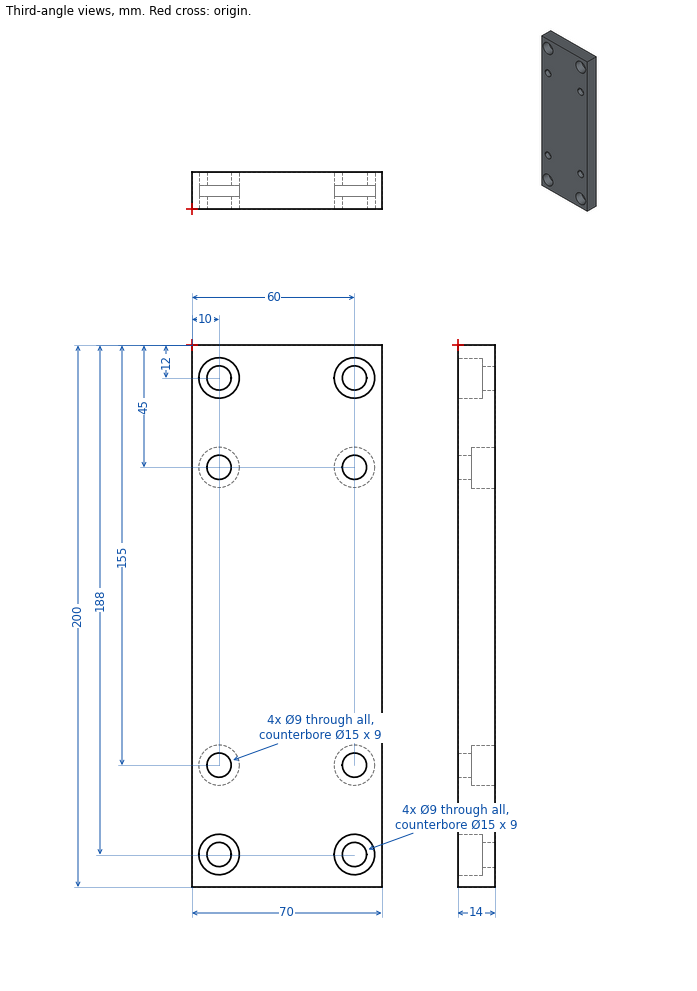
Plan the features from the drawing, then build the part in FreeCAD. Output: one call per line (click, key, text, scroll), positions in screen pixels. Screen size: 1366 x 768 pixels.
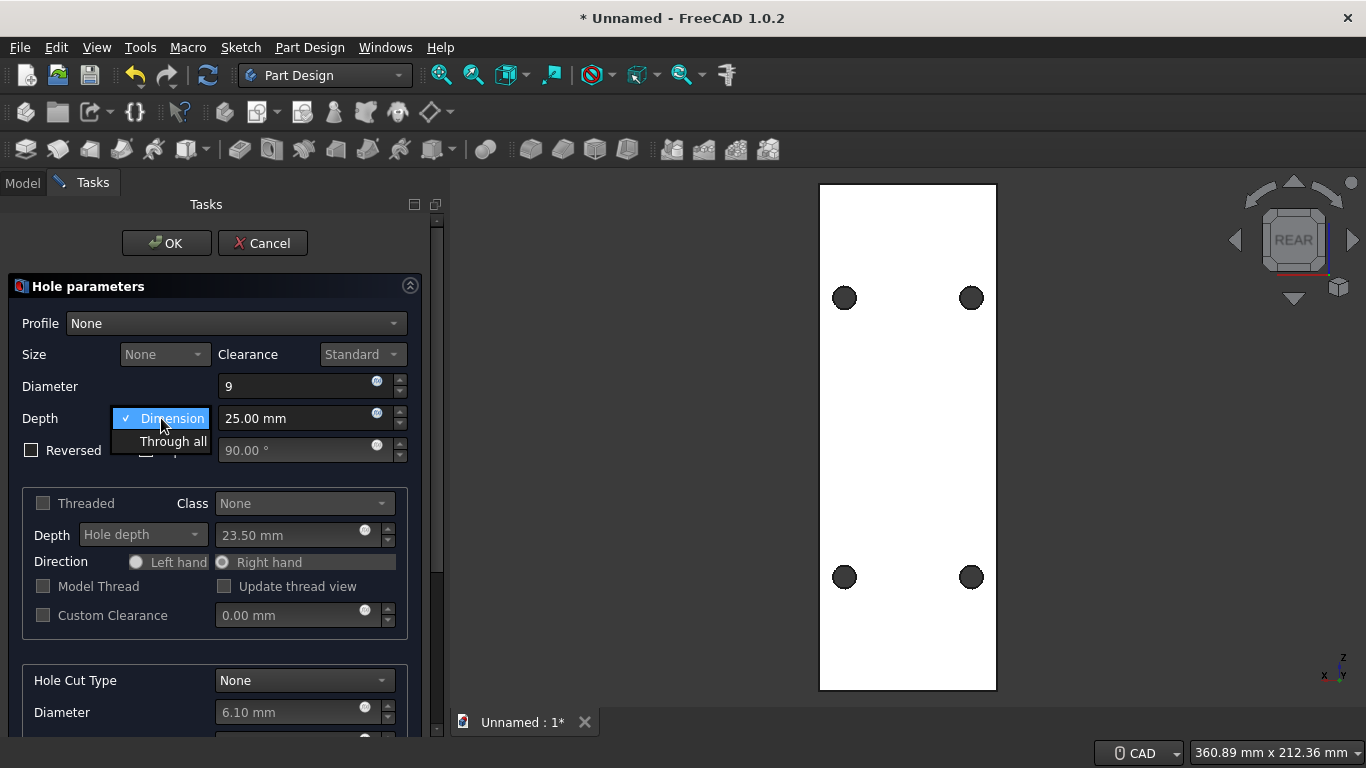
click(160, 442)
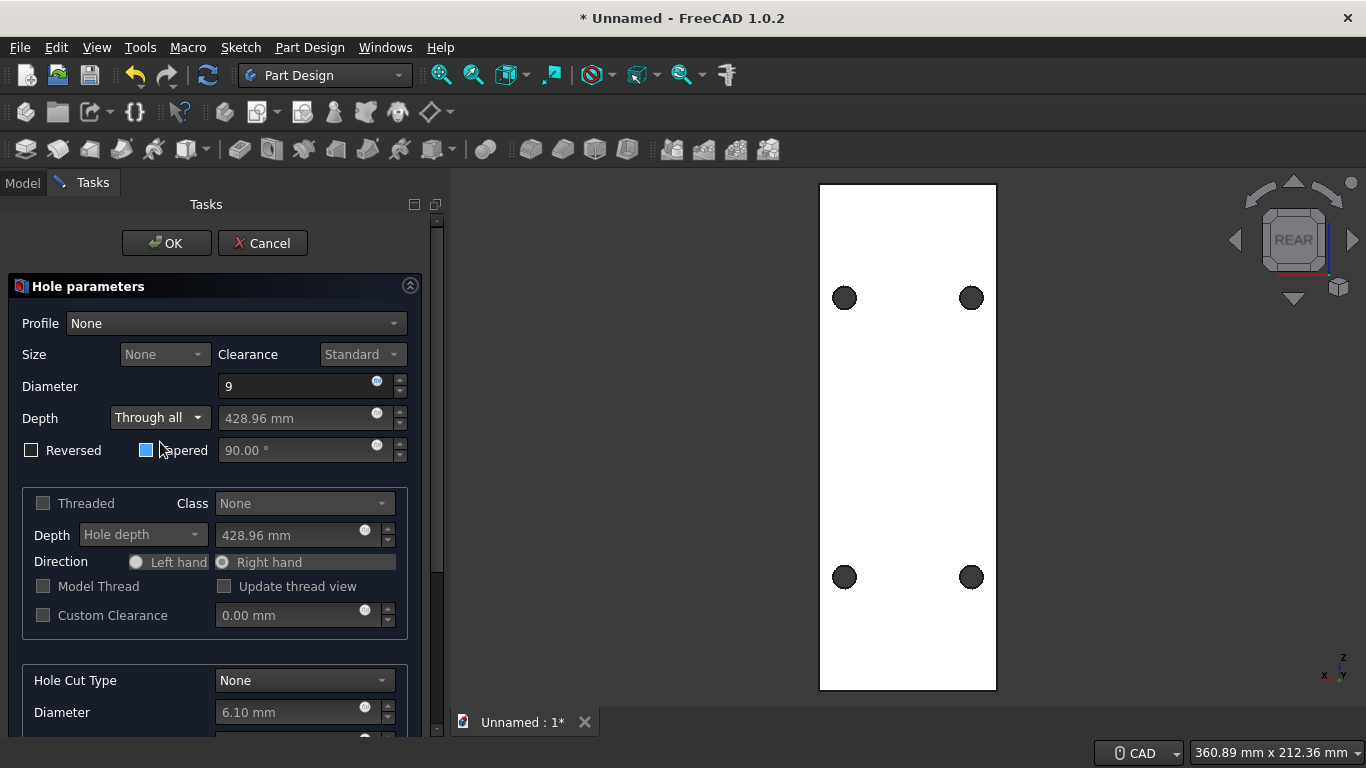
click(306, 680)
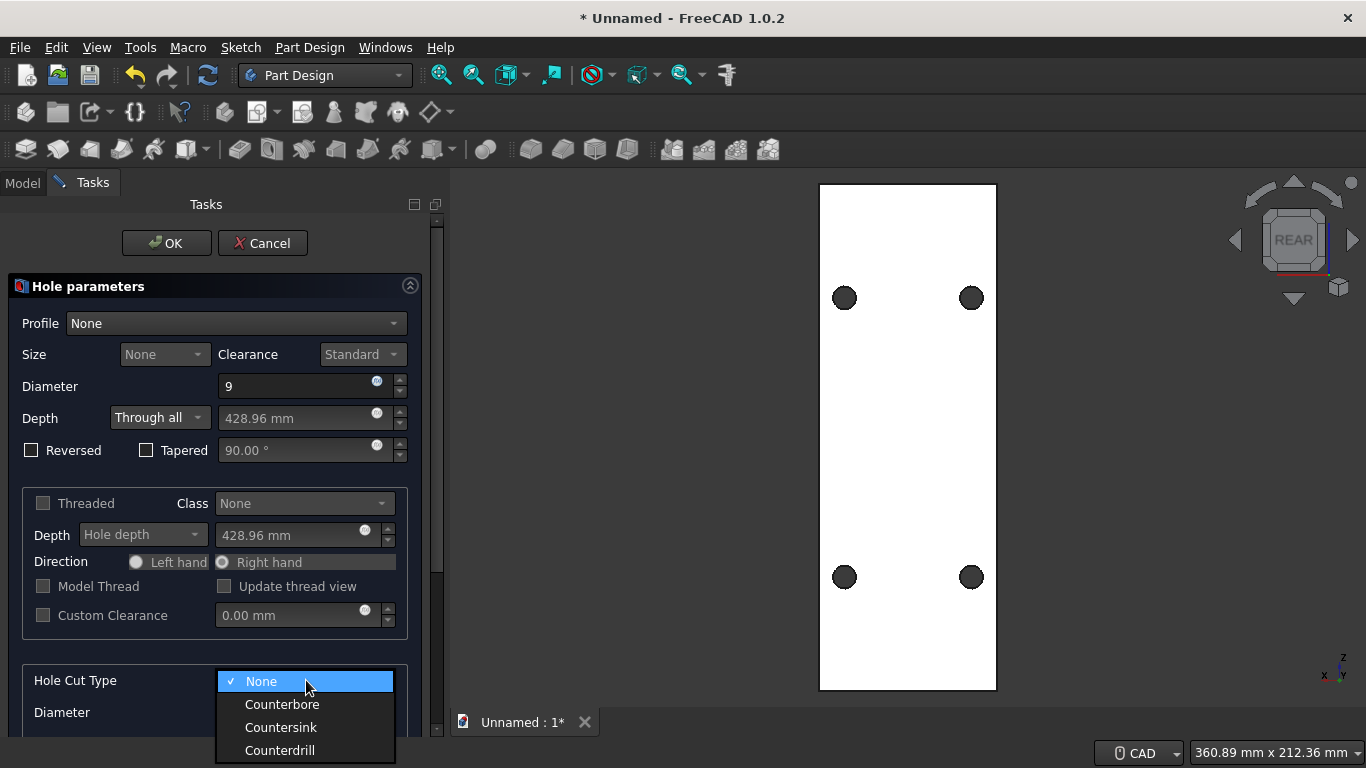
click(304, 704)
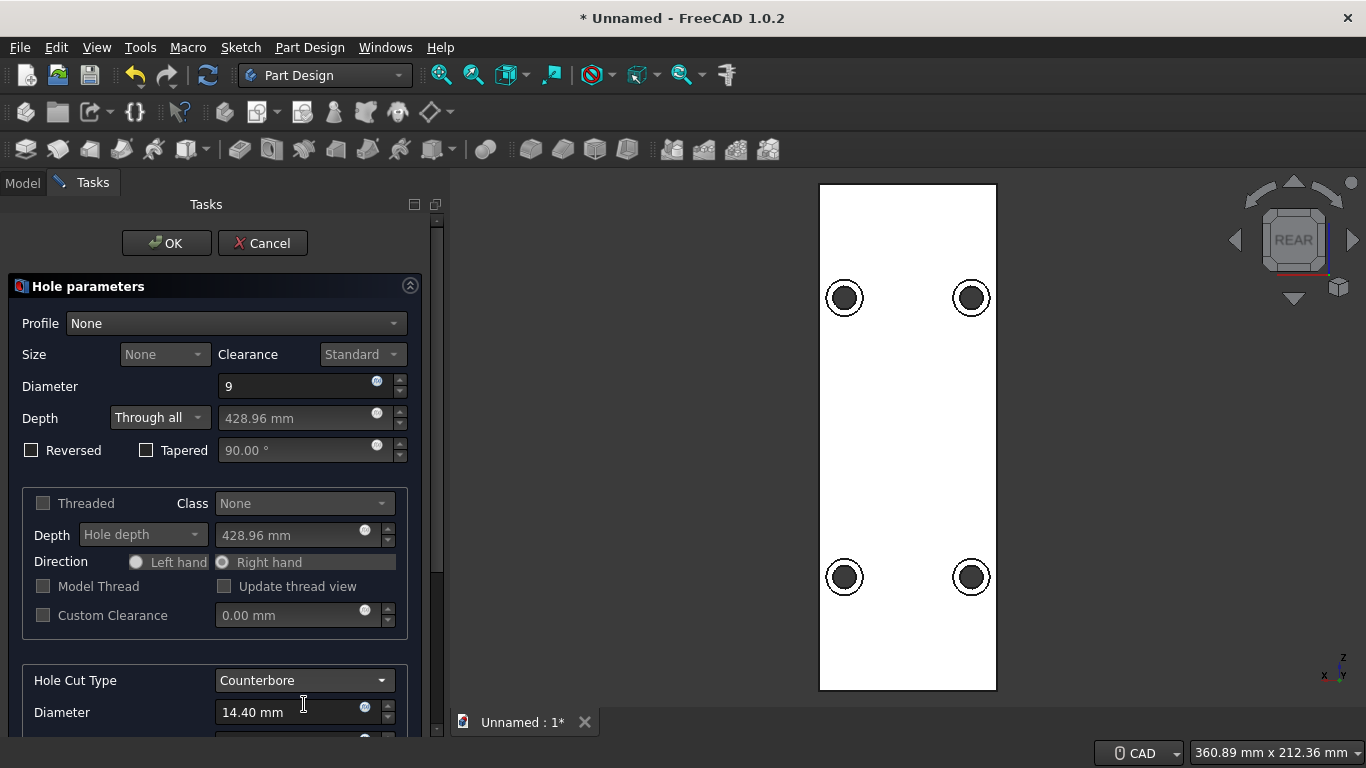
triple_click(298, 712)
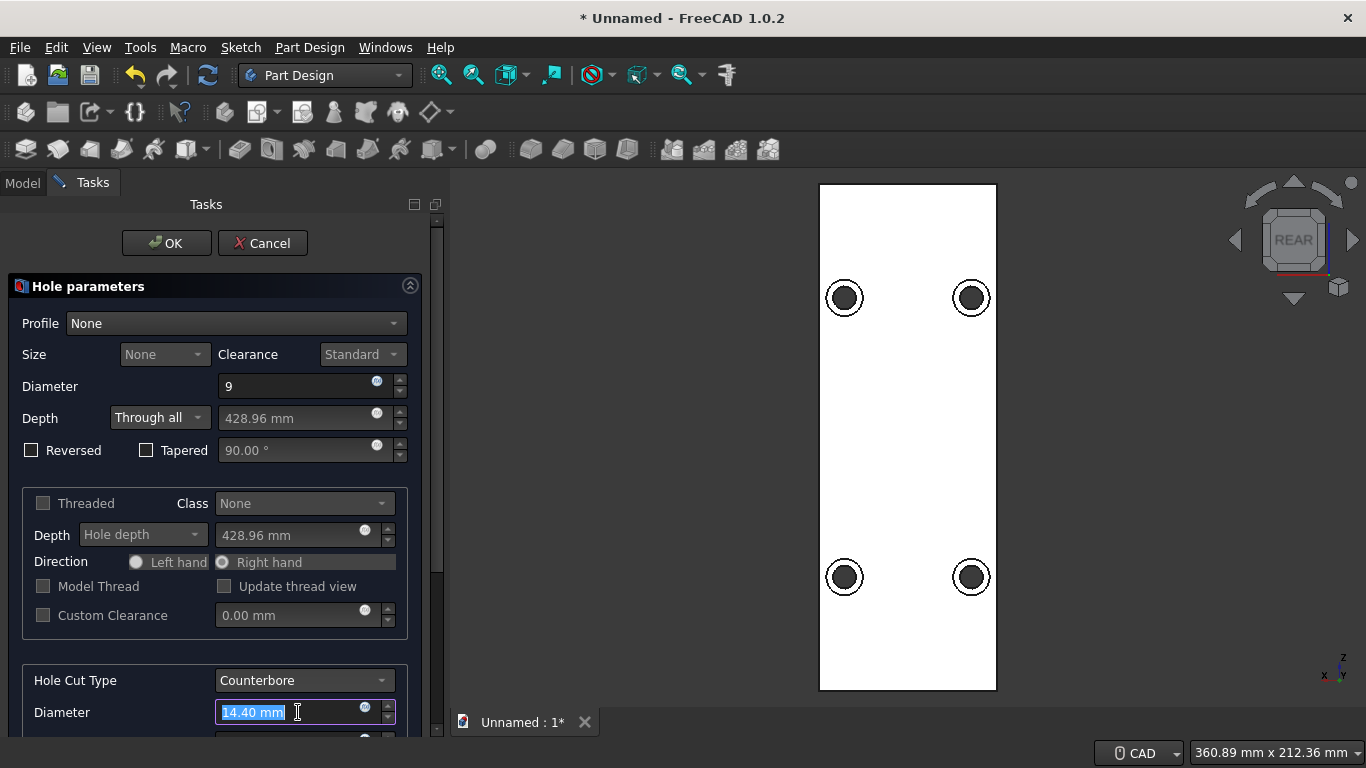
text(15)
key(Tab)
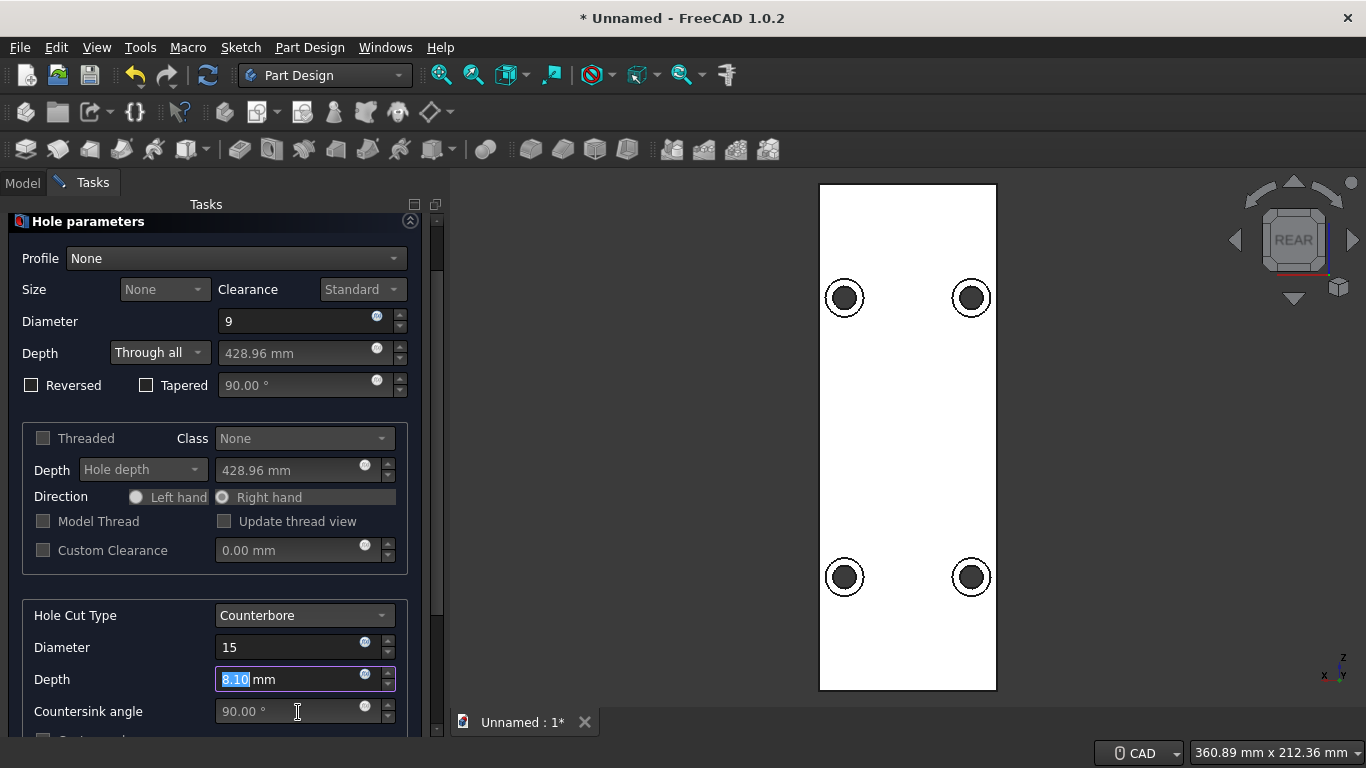
text(9)
key(Tab)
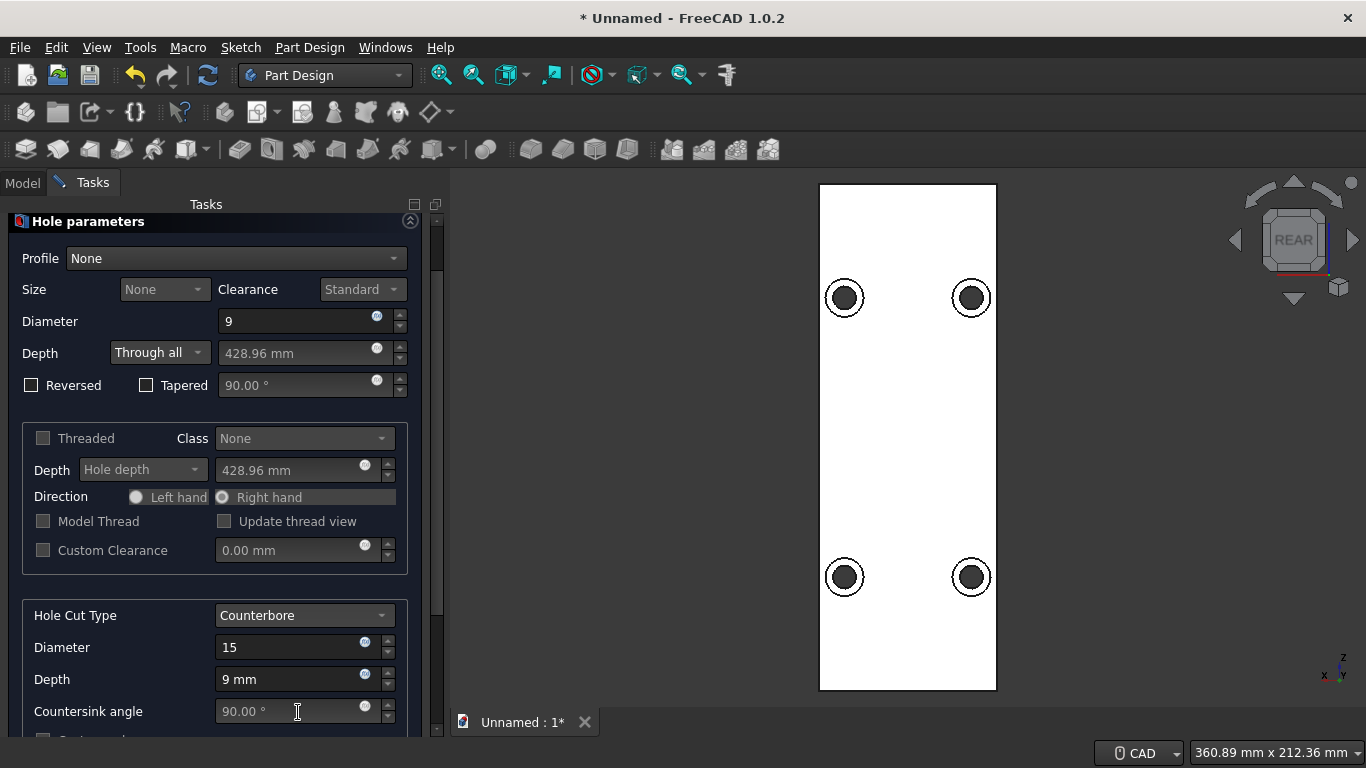
scroll(437, 475, up, 2)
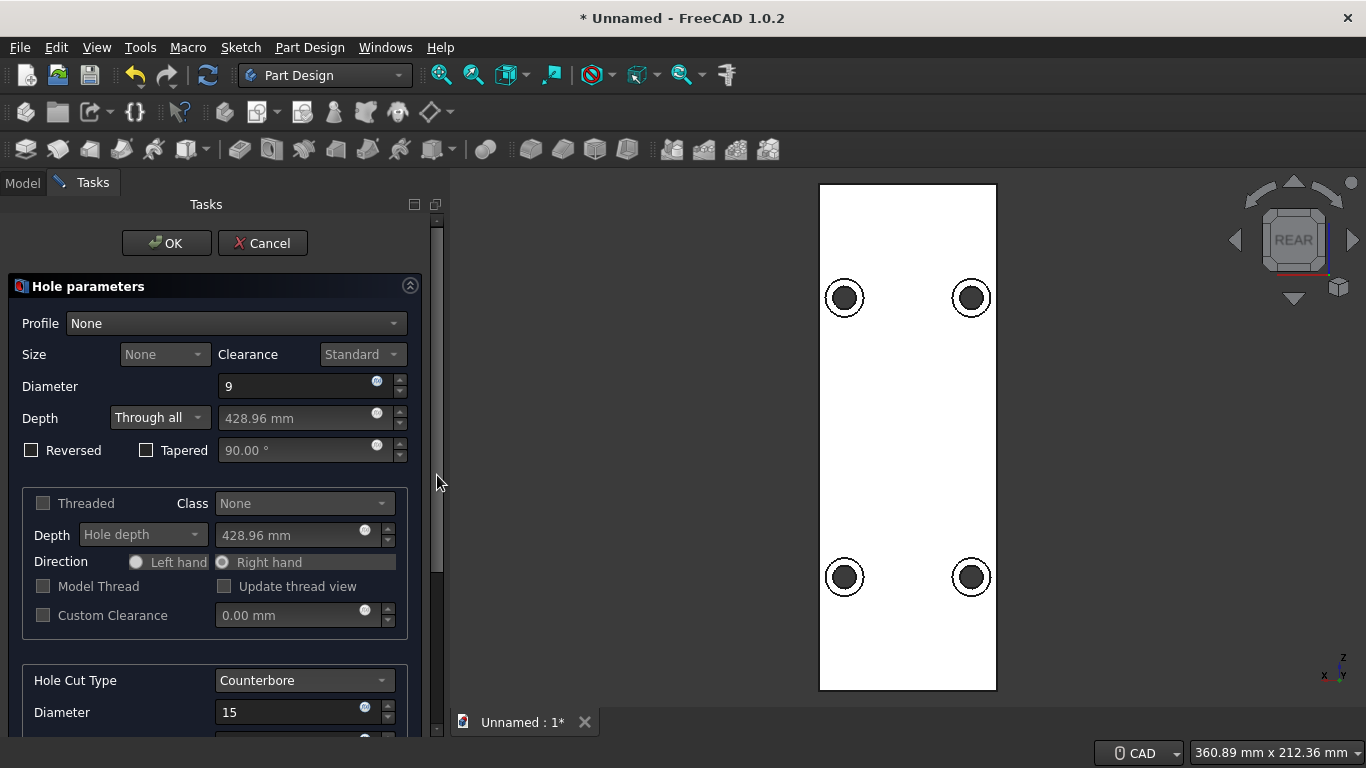
click(167, 243)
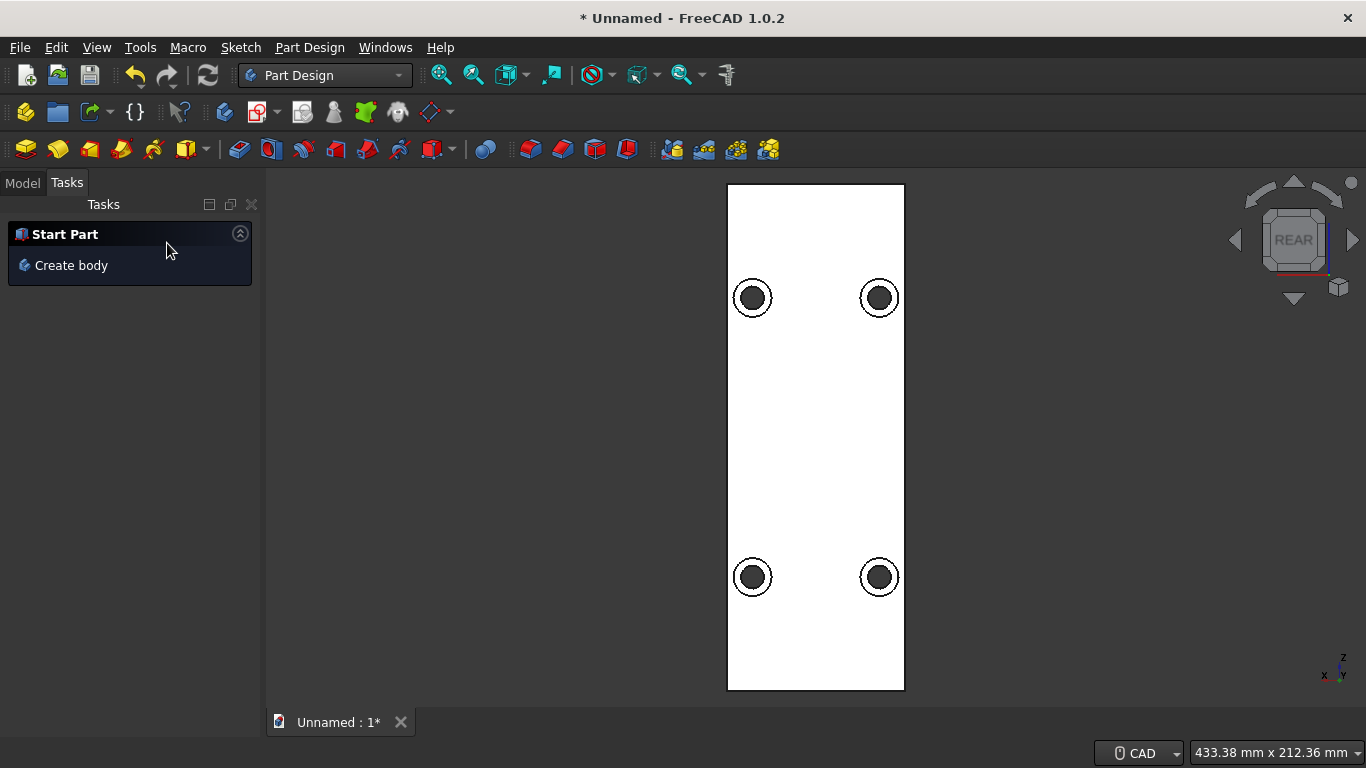
key(0)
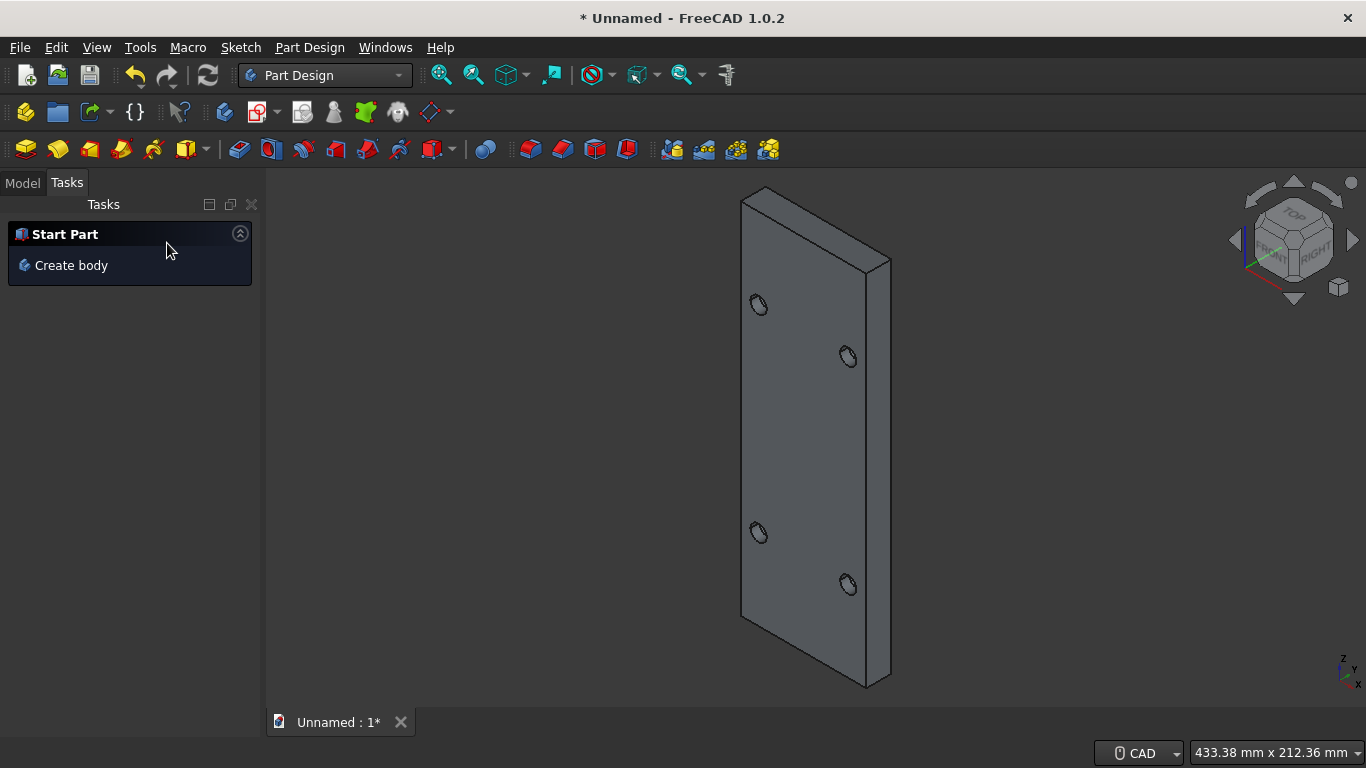
click(803, 444)